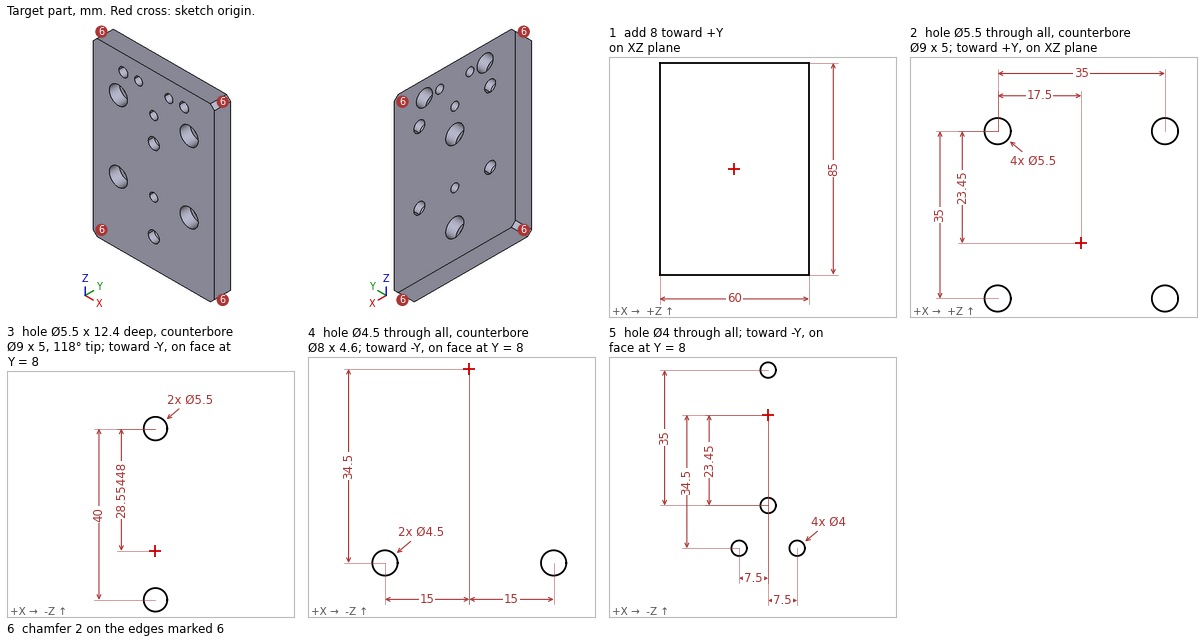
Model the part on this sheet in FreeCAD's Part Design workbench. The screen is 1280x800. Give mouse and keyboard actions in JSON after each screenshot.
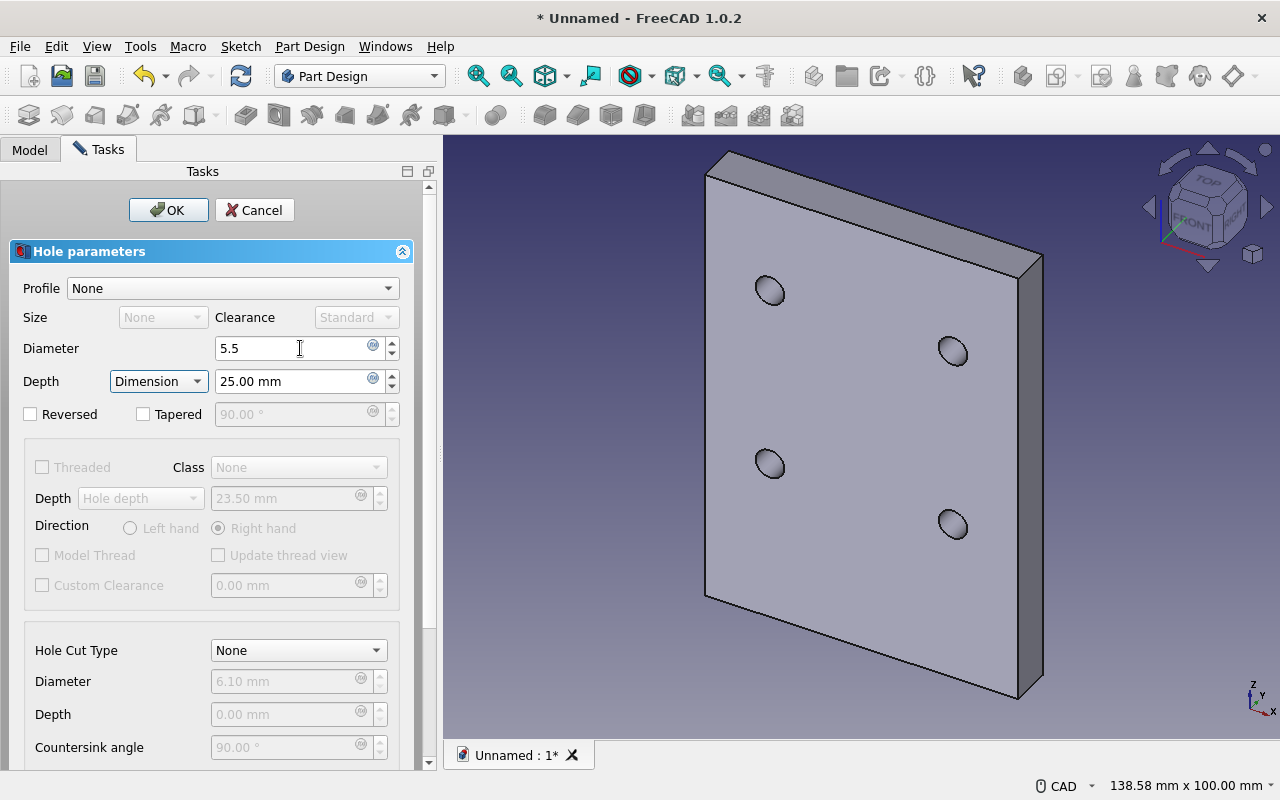
{"action": "left_click", "coordinate": [160, 382]}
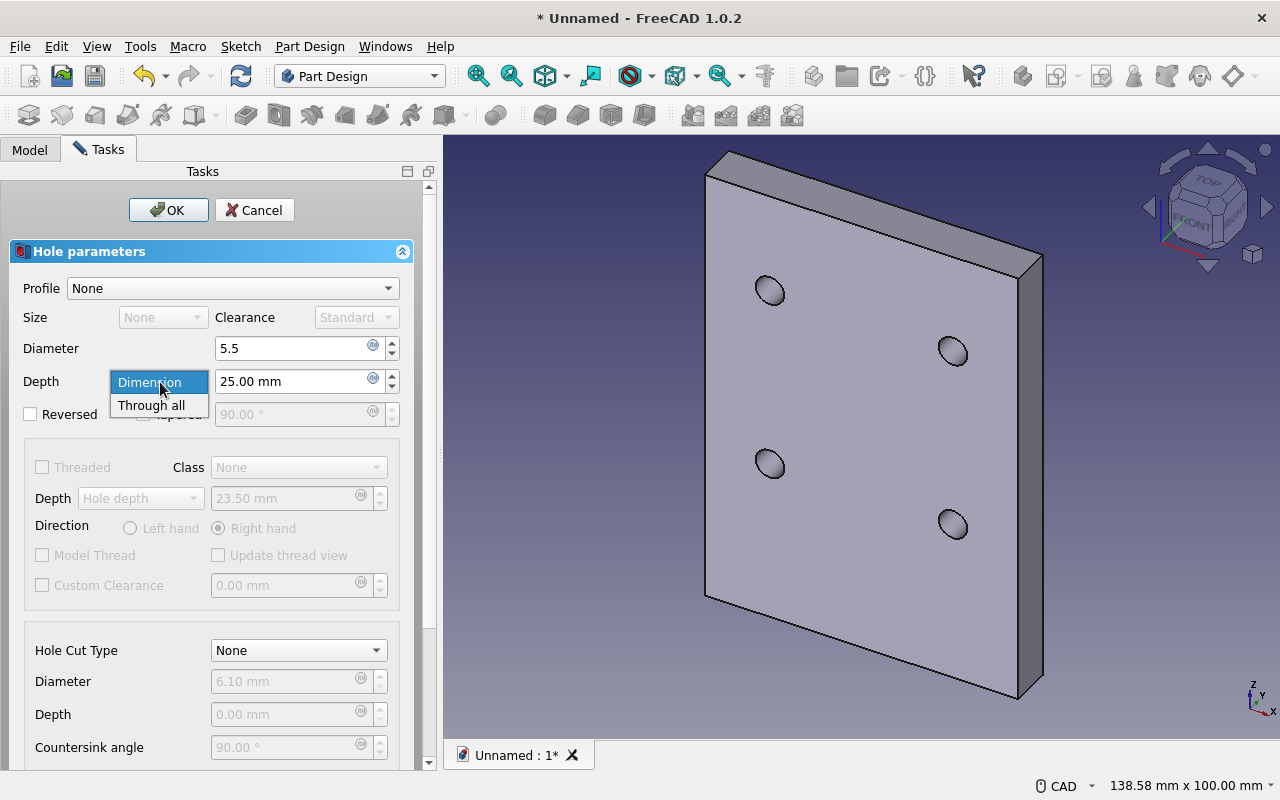
{"action": "left_click", "coordinate": [158, 406]}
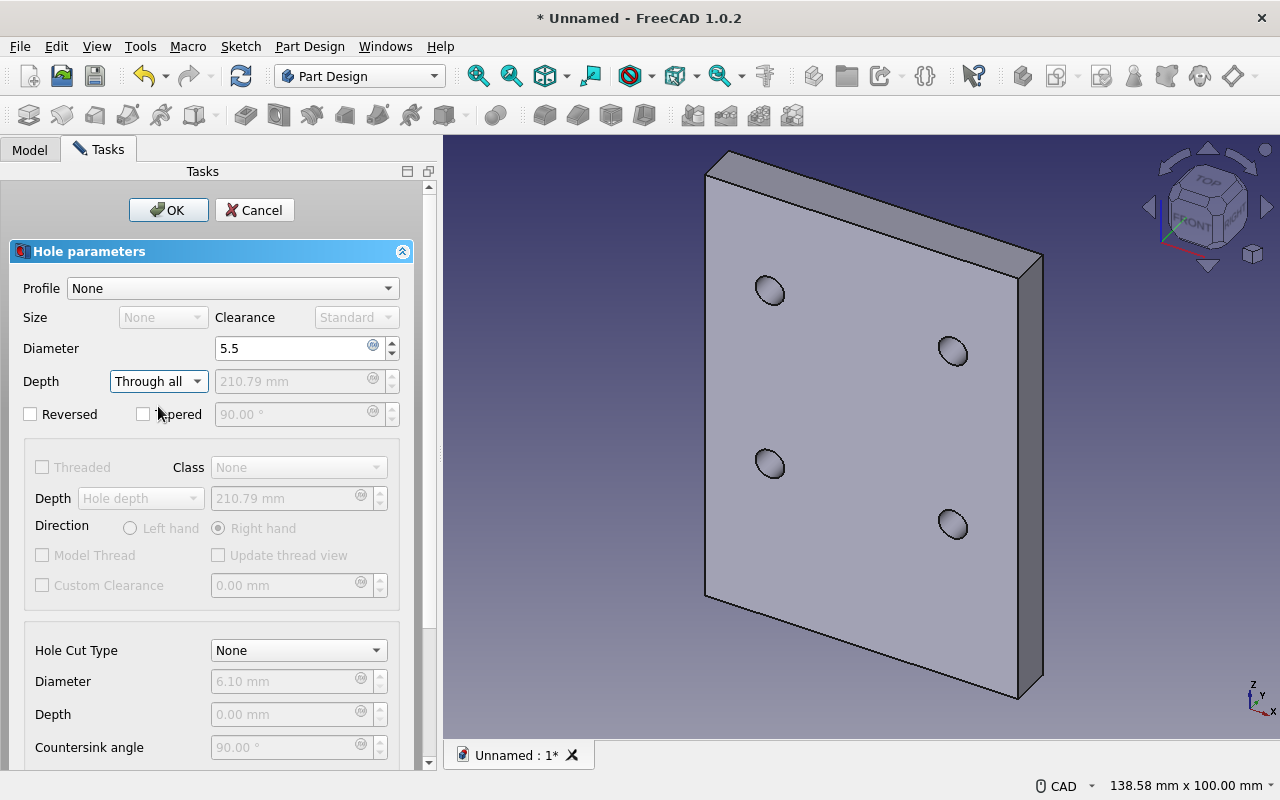
{"action": "left_click", "coordinate": [300, 650]}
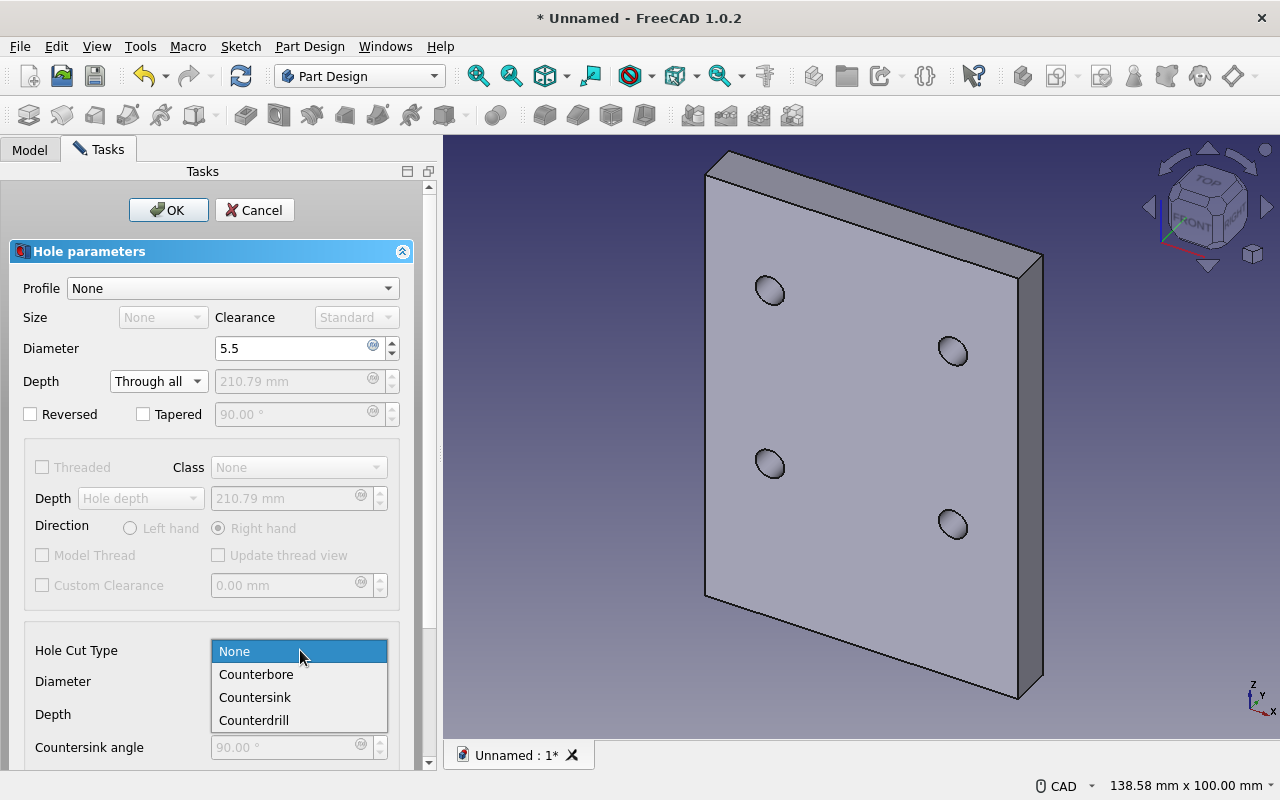
{"action": "left_click", "coordinate": [298, 674]}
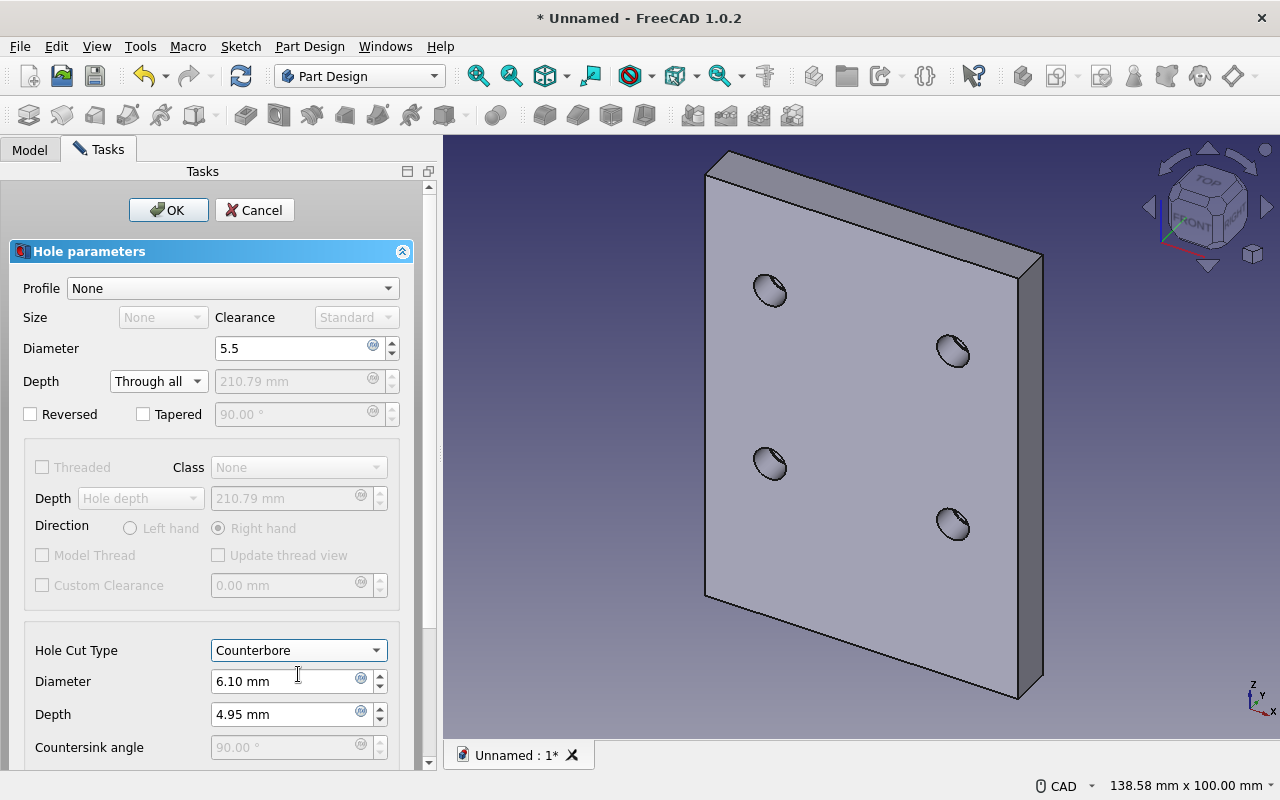
{"action": "triple_click", "coordinate": [292, 682]}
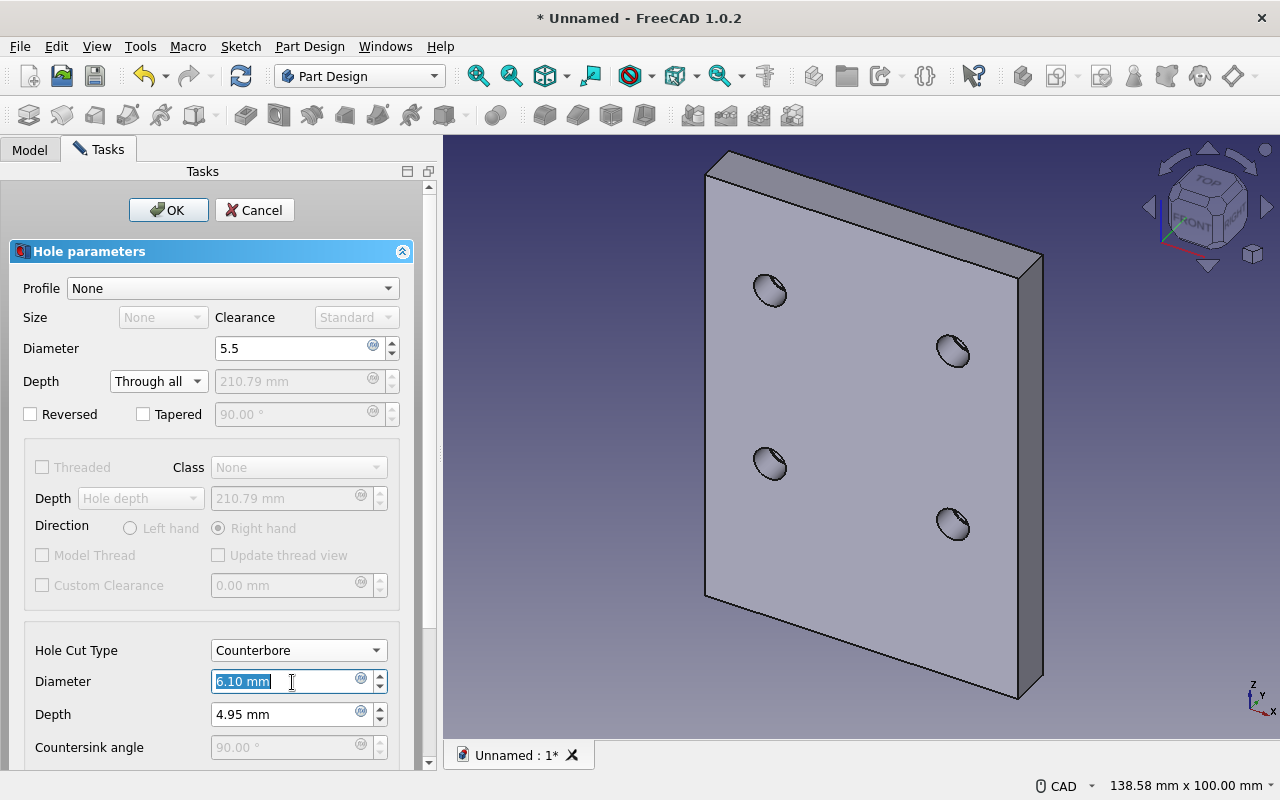
{"action": "type", "text": "9"}
{"action": "key", "text": "Tab"}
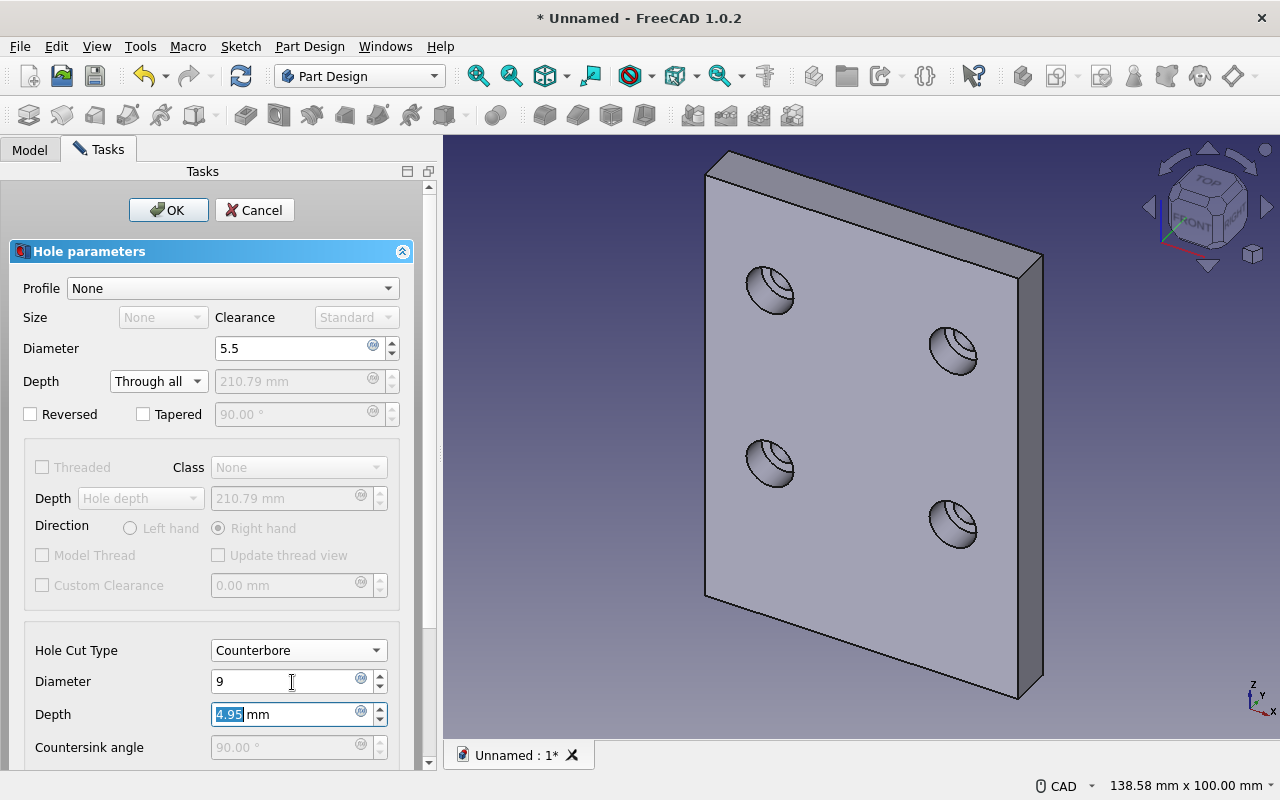
{"action": "type", "text": "5"}
{"action": "key", "text": "Tab"}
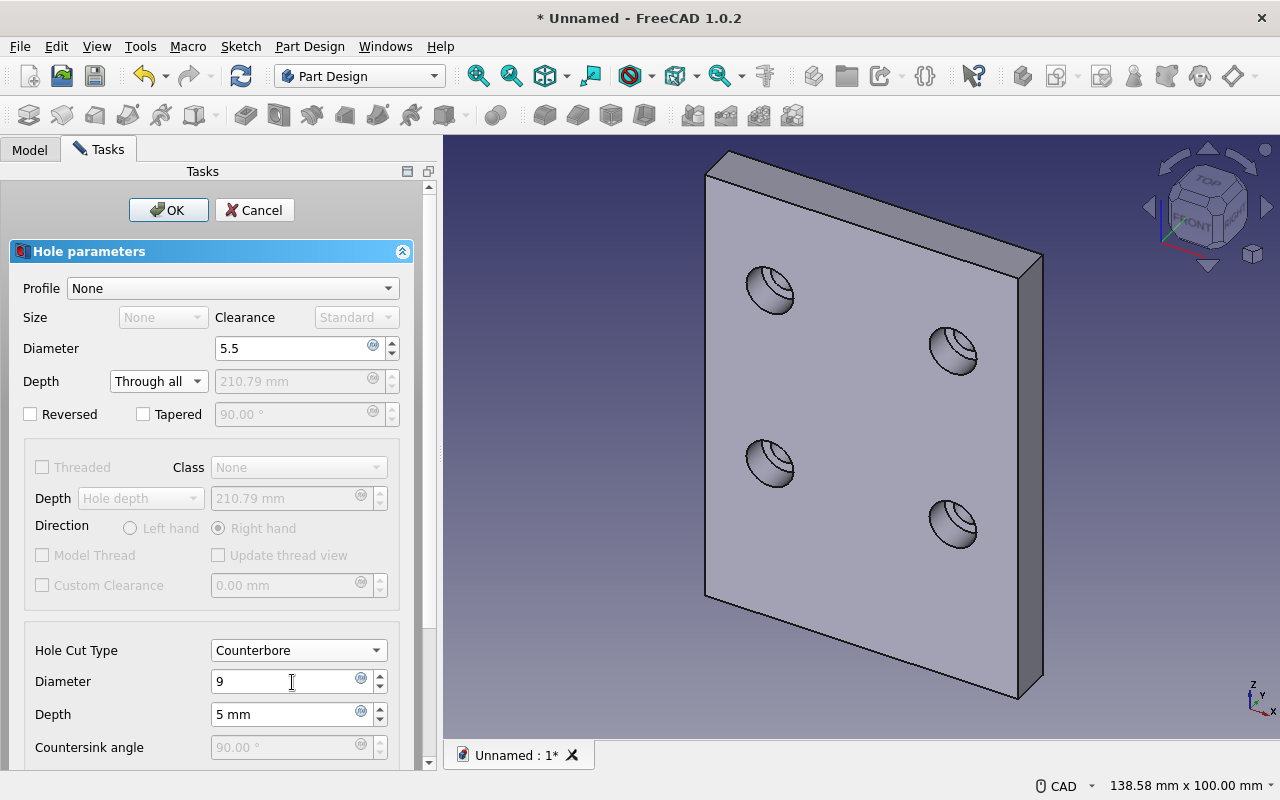
{"action": "left_click", "coordinate": [169, 210]}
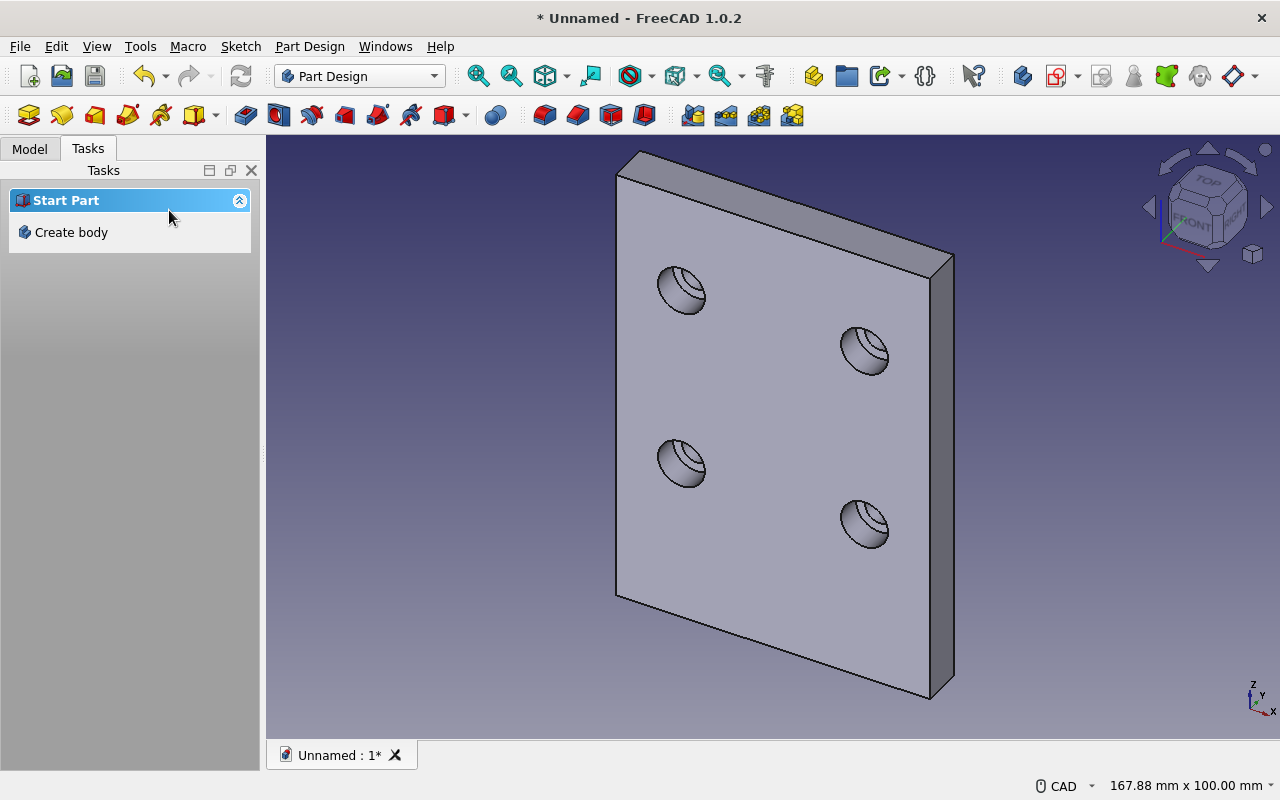
{"action": "key", "text": "4"}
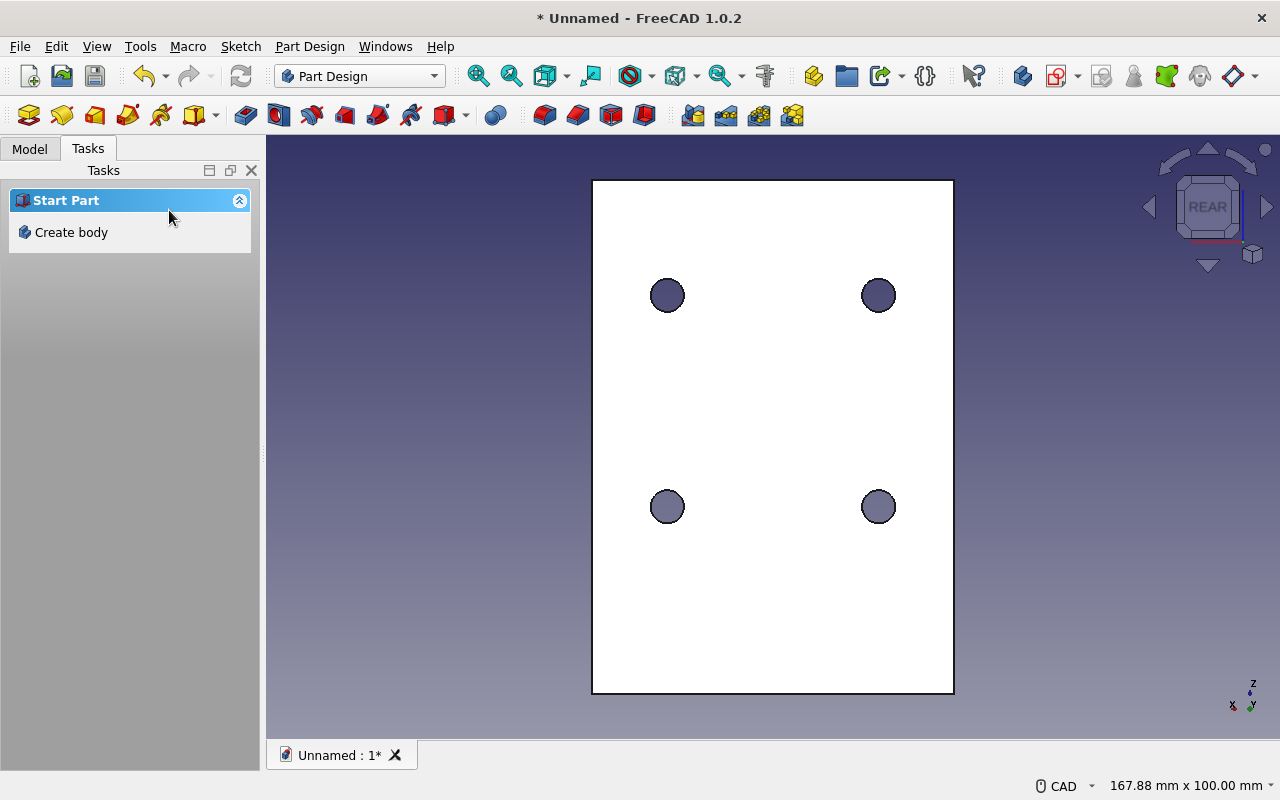
{"action": "left_click", "coordinate": [773, 436]}